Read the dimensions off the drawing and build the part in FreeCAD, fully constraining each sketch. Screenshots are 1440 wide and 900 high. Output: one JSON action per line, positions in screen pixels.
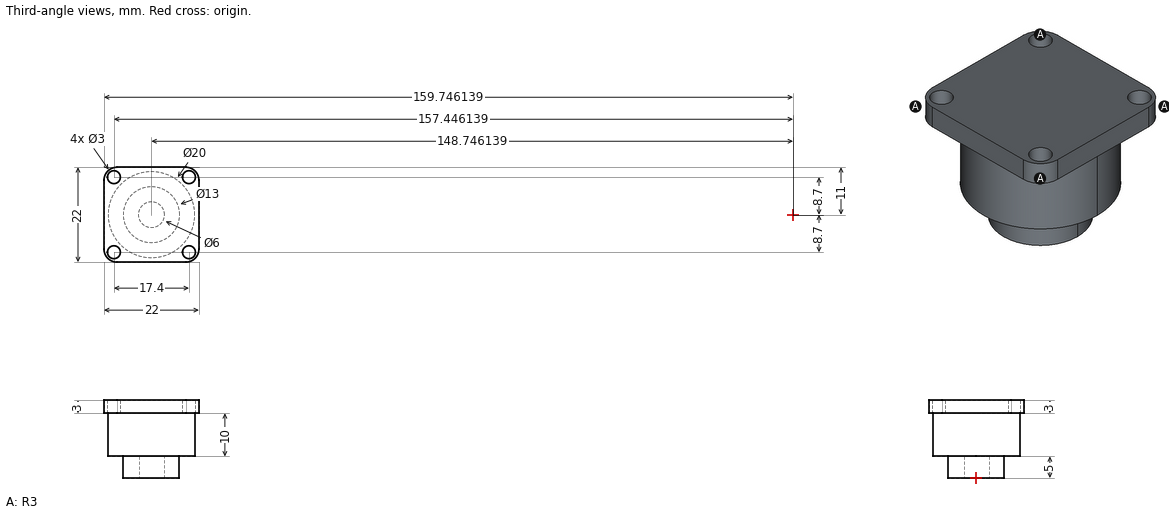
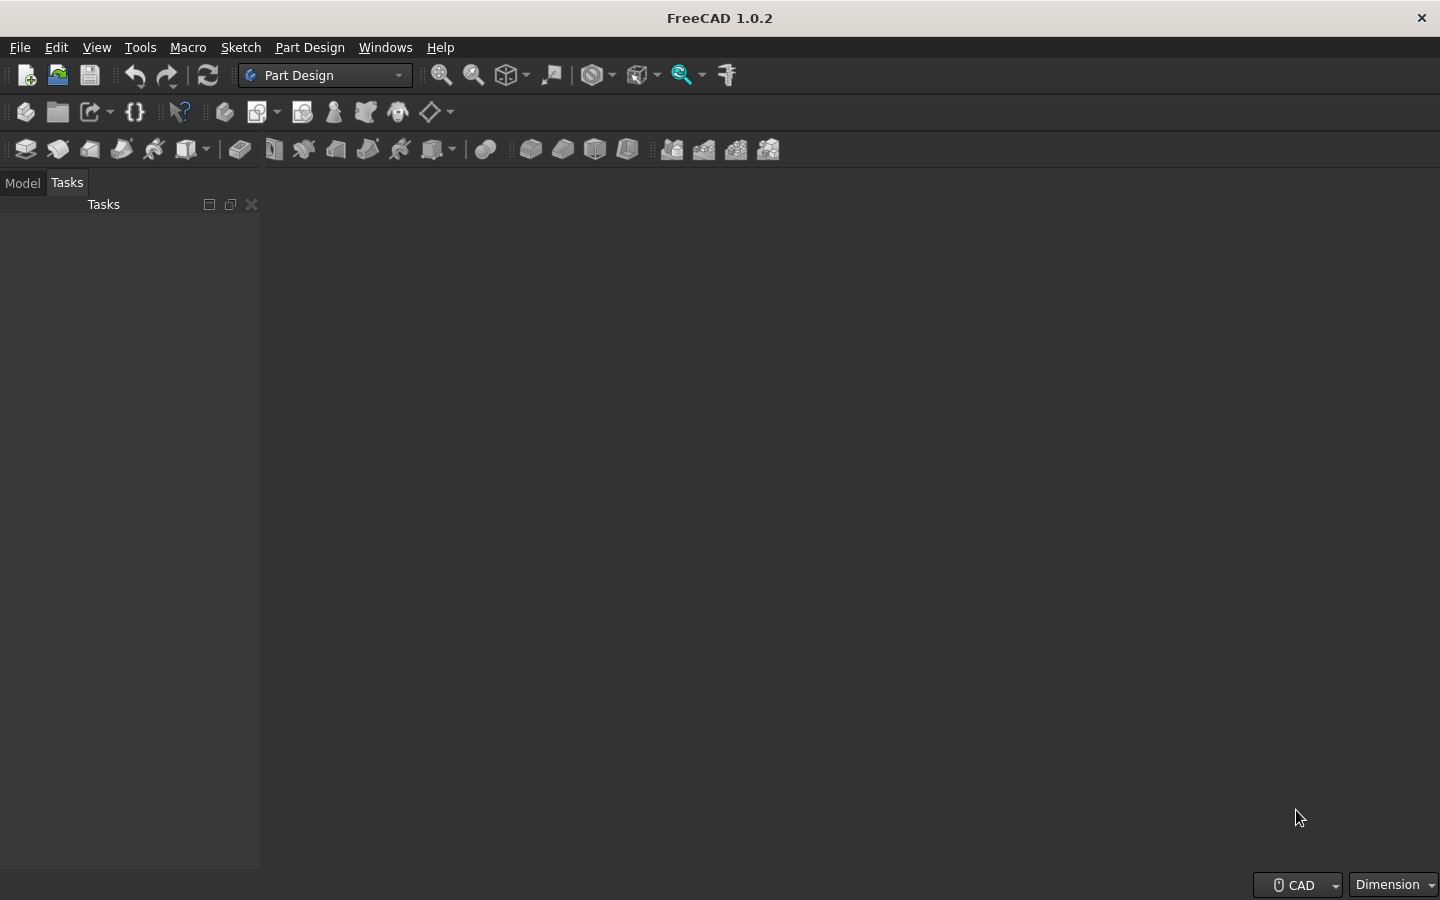
{"action": "left_click", "coordinate": [1288, 76]}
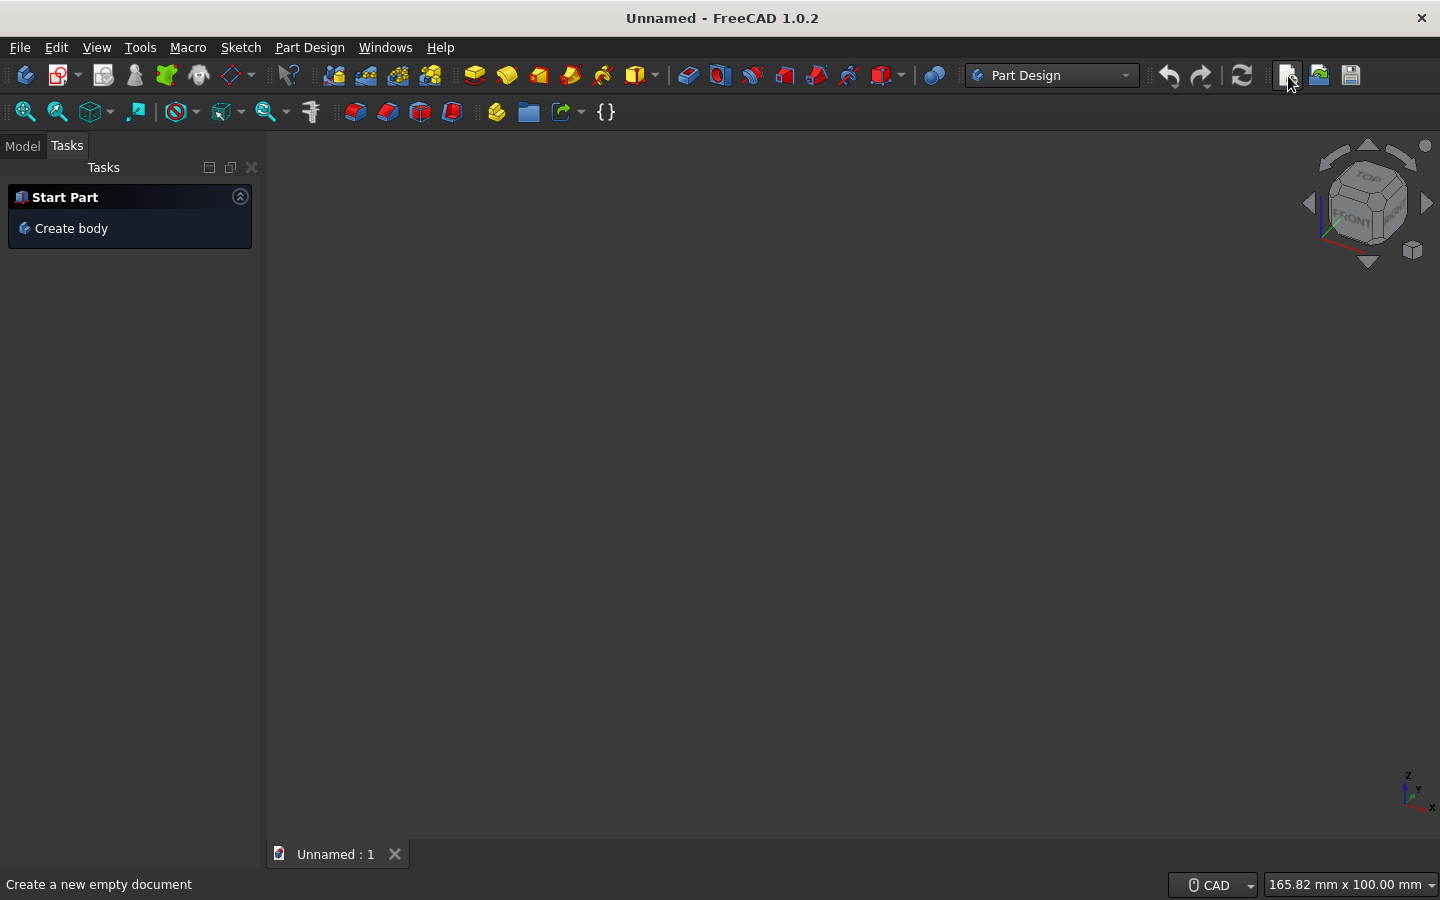
{"action": "left_click", "coordinate": [58, 76]}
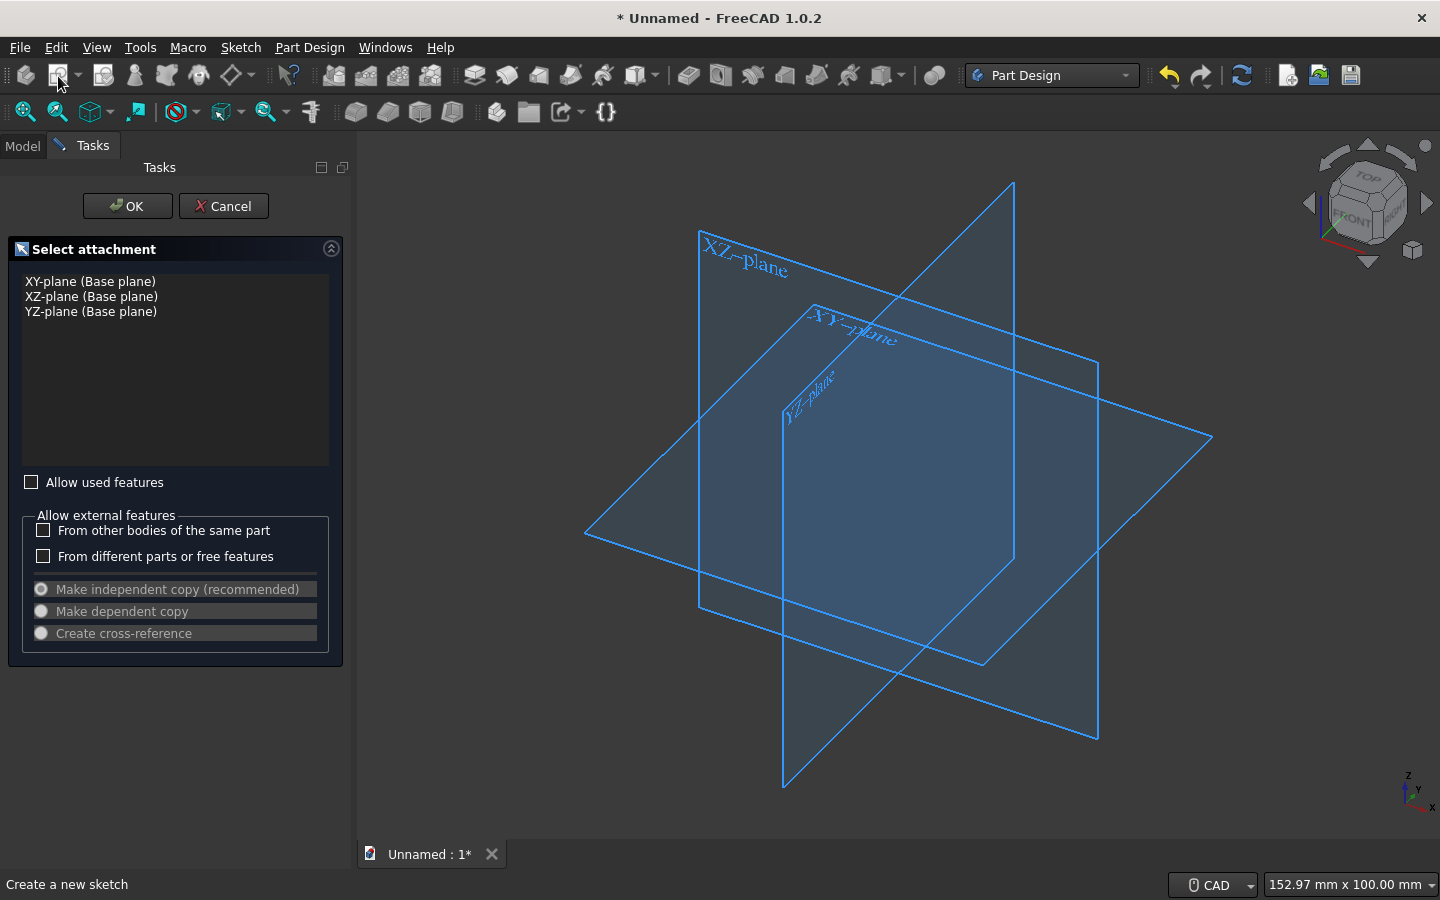
{"action": "left_click", "coordinate": [82, 282]}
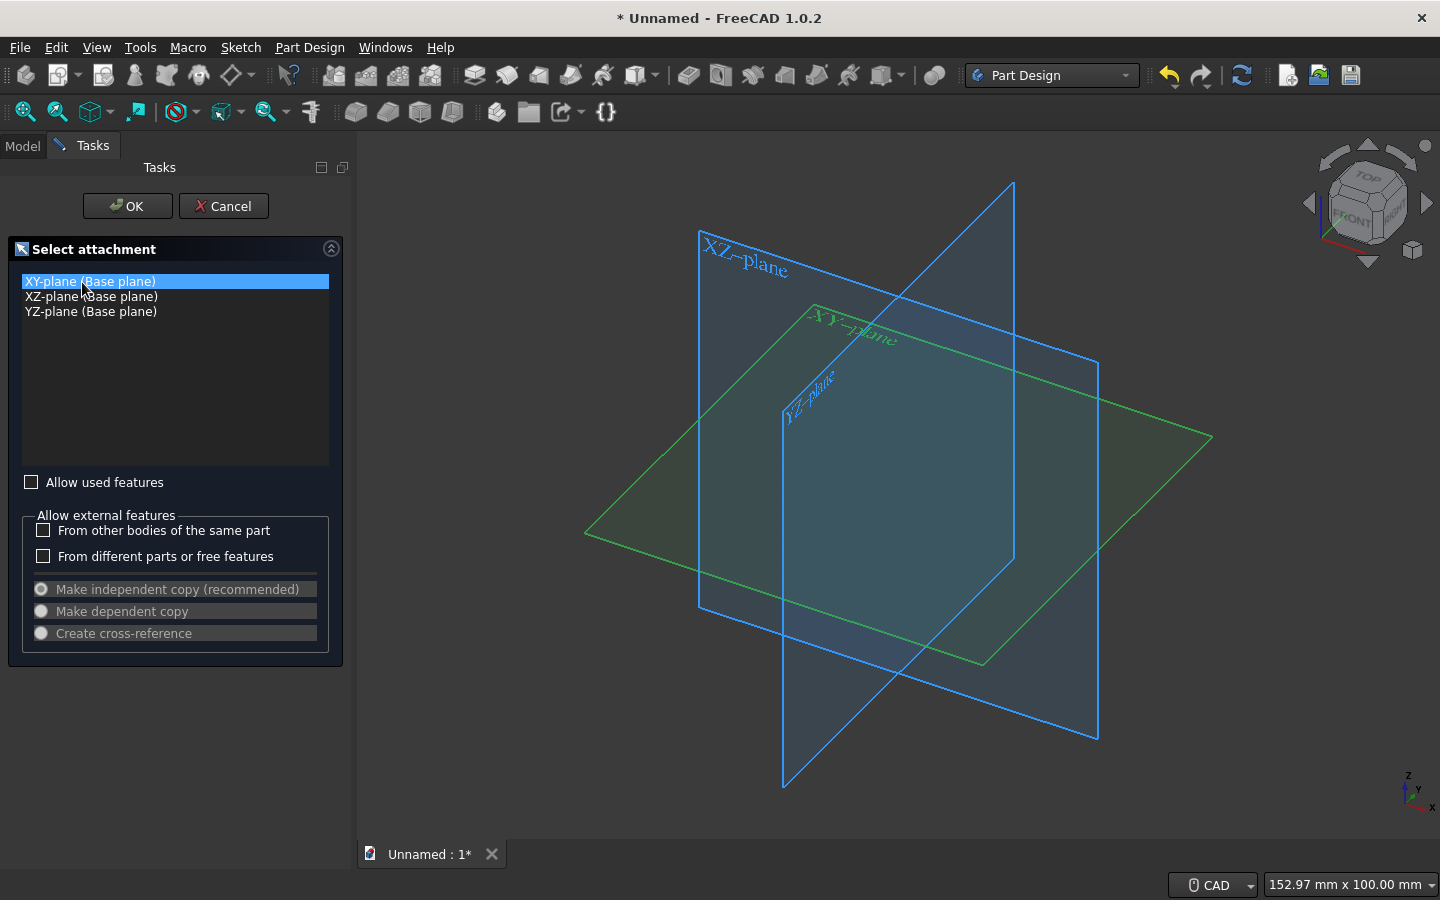
{"action": "left_click", "coordinate": [128, 206]}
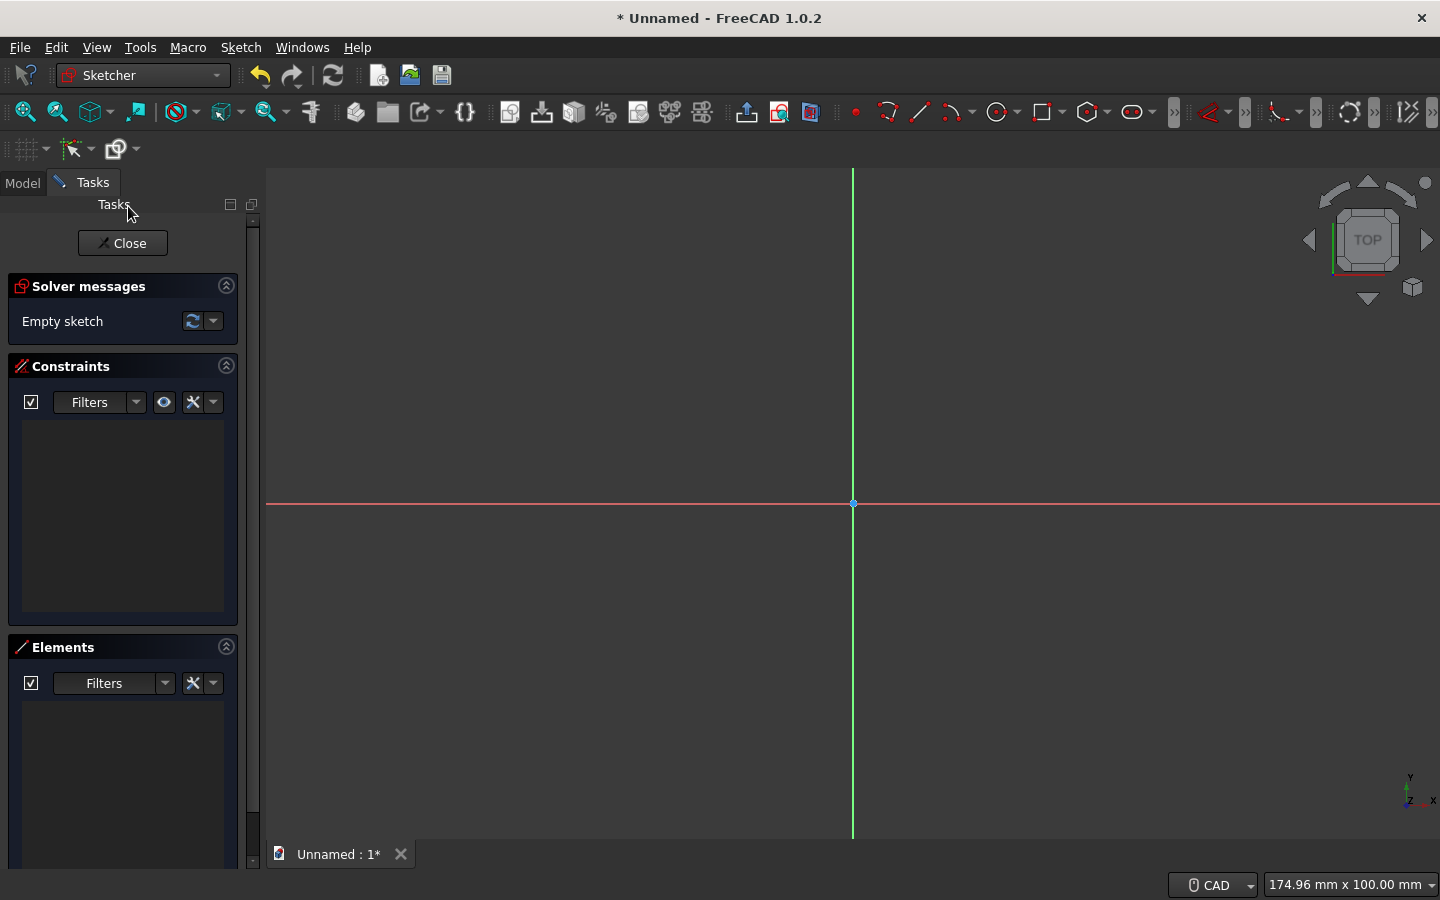
{"action": "scroll", "coordinate": [784, 504], "scroll_direction": "down", "scroll_amount": 5}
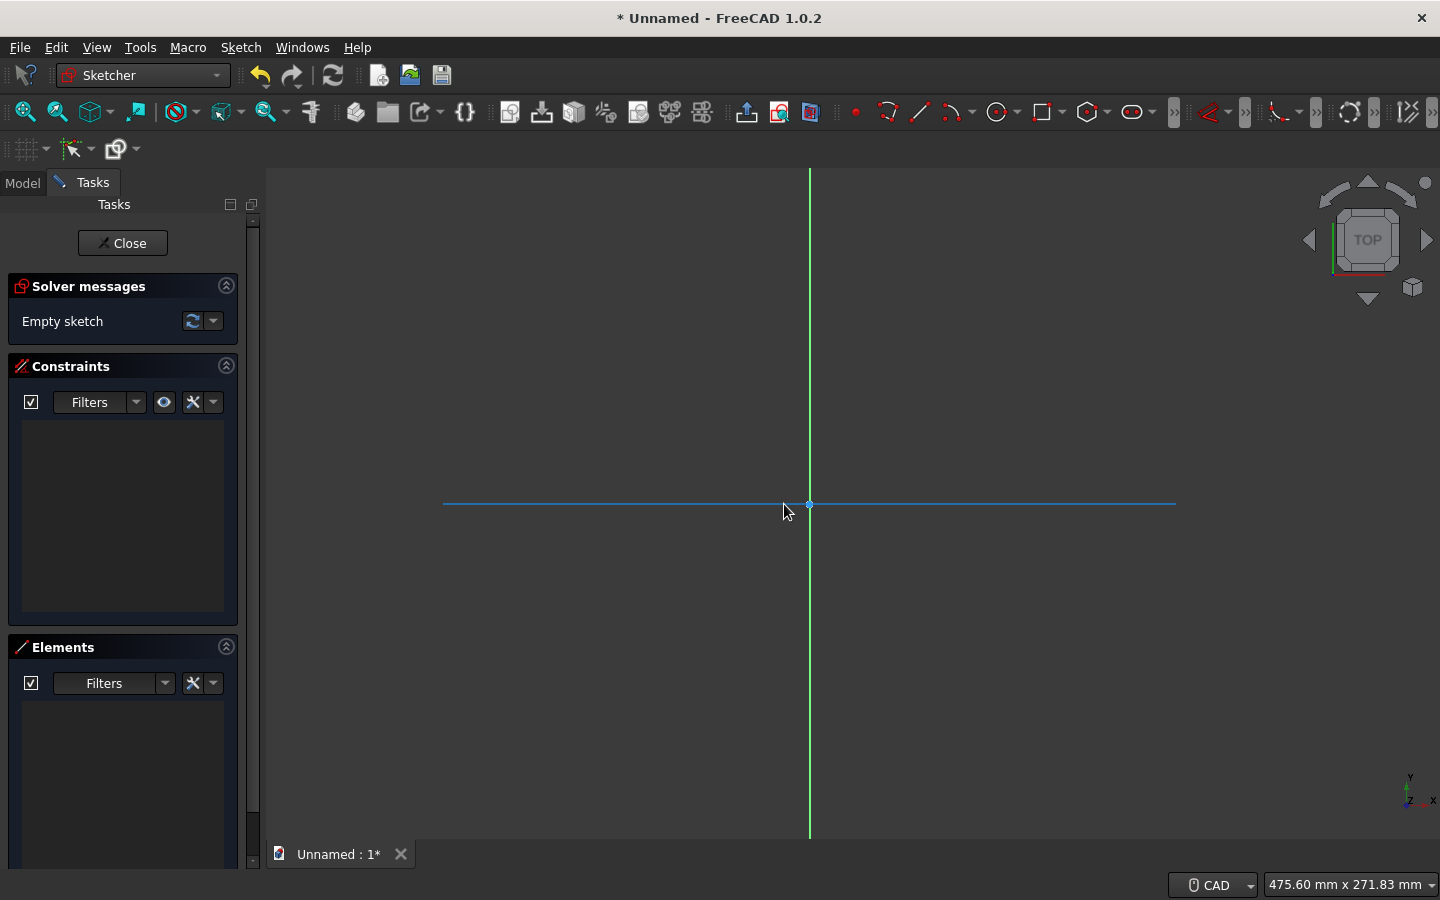
{"action": "scroll", "coordinate": [415, 504], "scroll_direction": "up", "scroll_amount": 13}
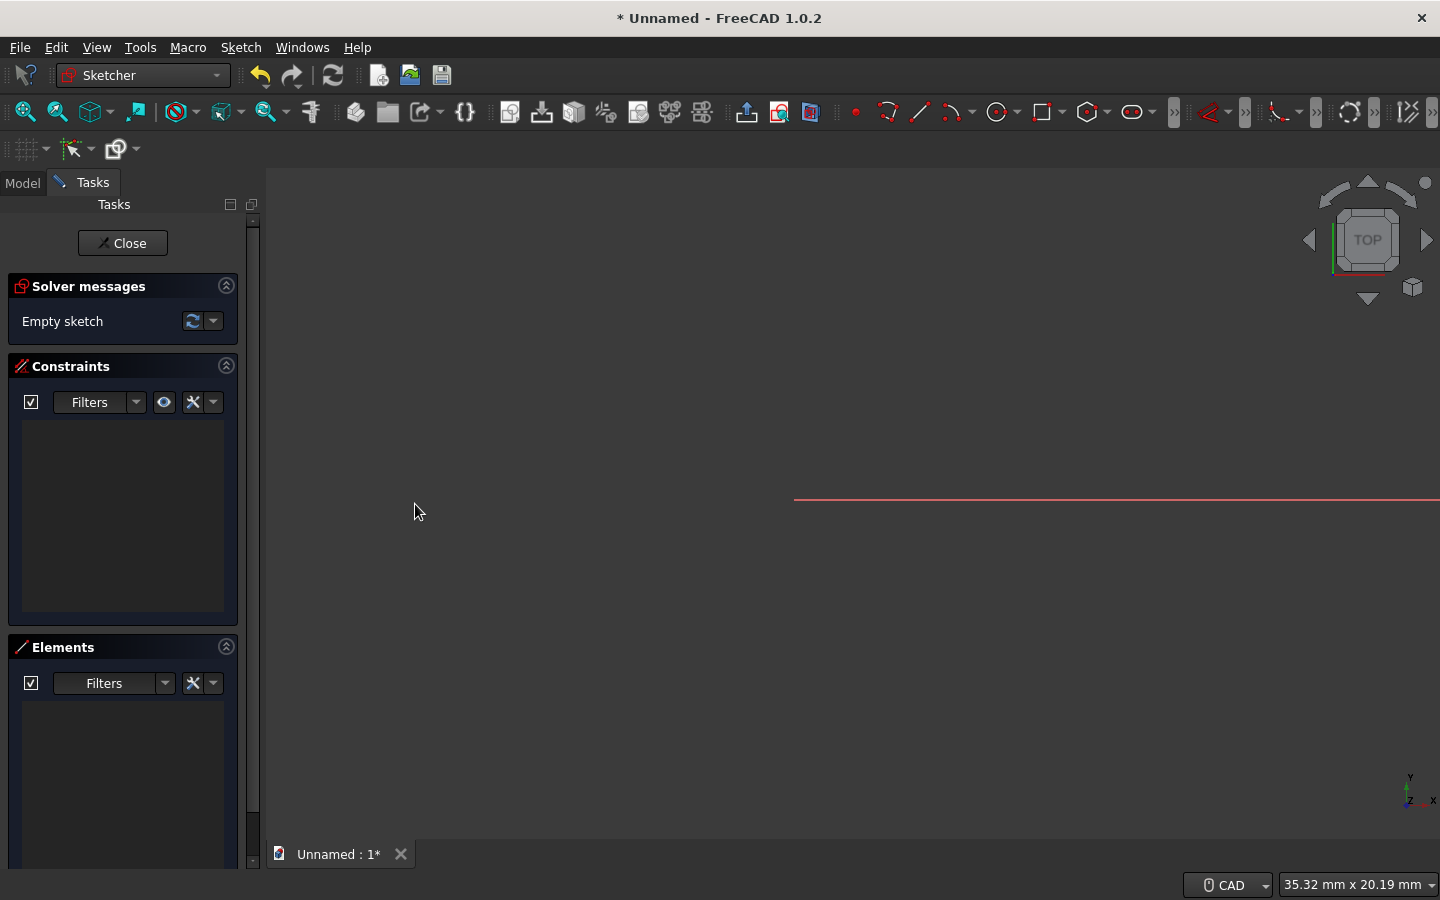
{"action": "key", "text": "g c"}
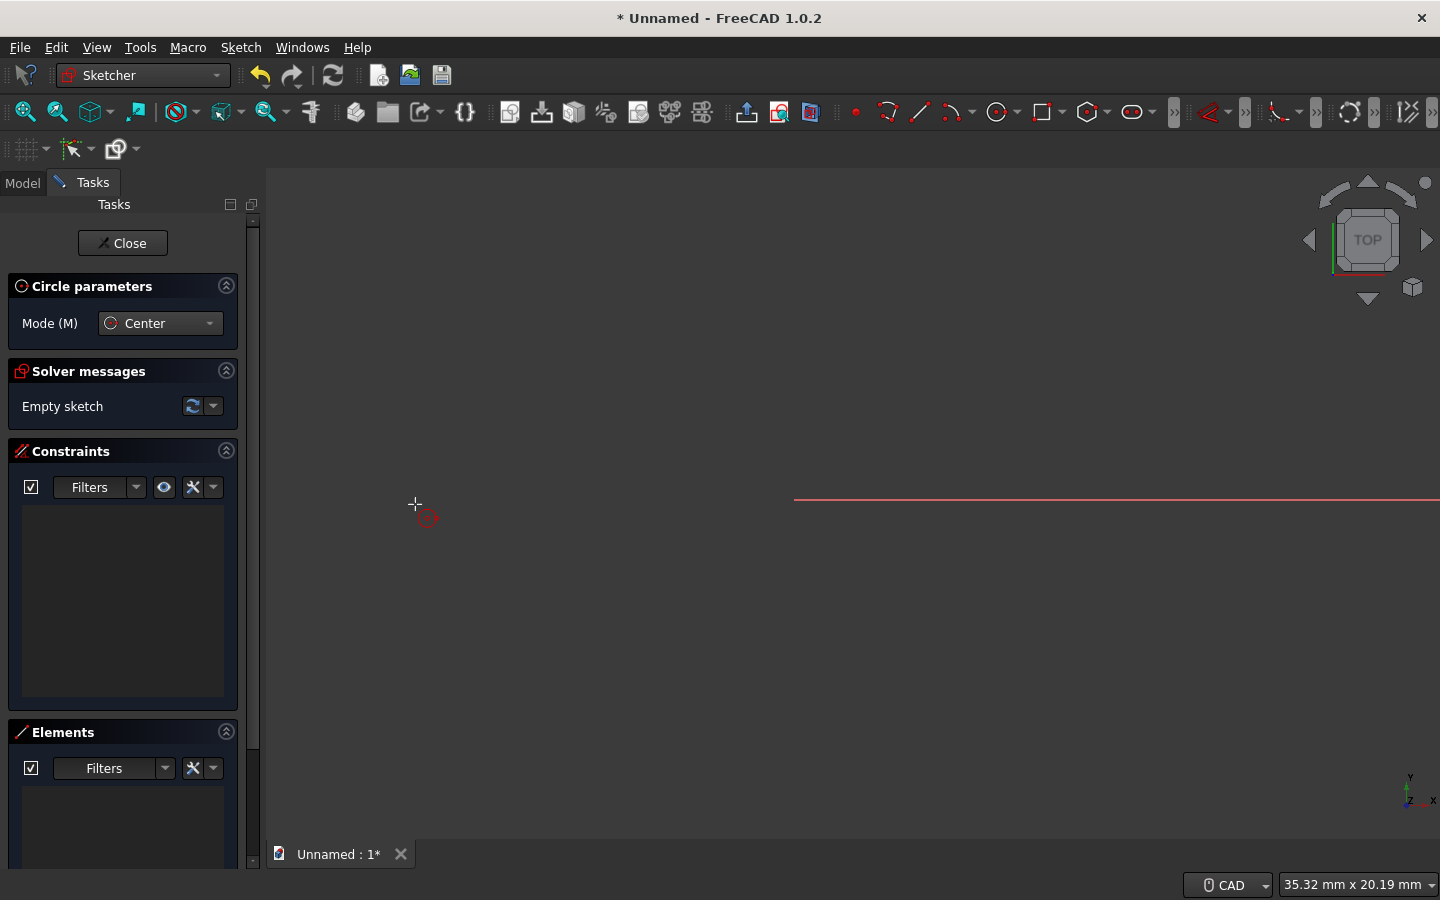
{"action": "left_click", "coordinate": [783, 500]}
{"action": "mouse_move", "coordinate": [936, 347]}